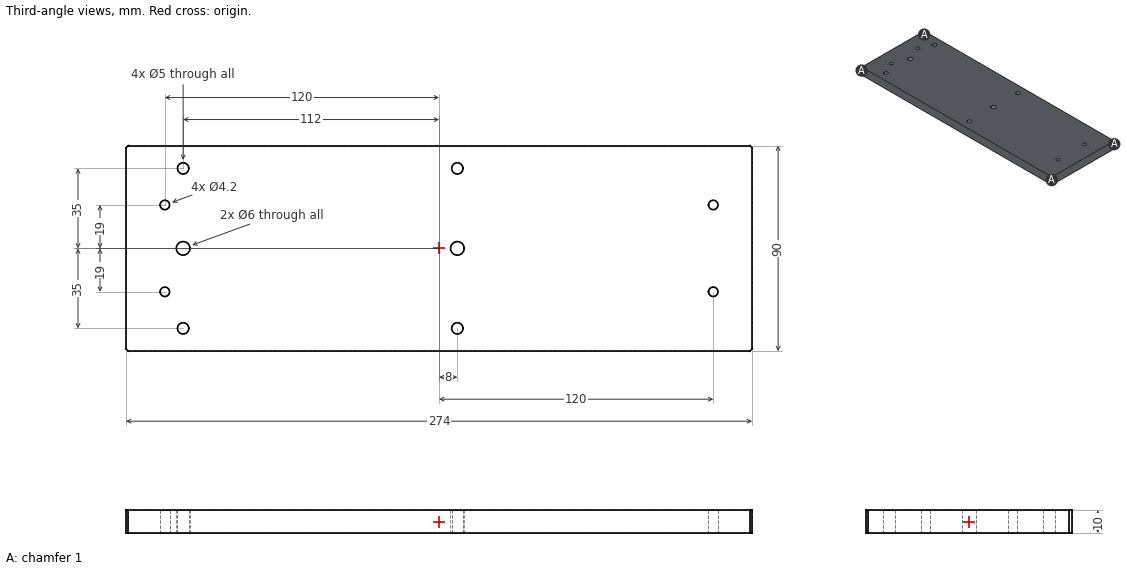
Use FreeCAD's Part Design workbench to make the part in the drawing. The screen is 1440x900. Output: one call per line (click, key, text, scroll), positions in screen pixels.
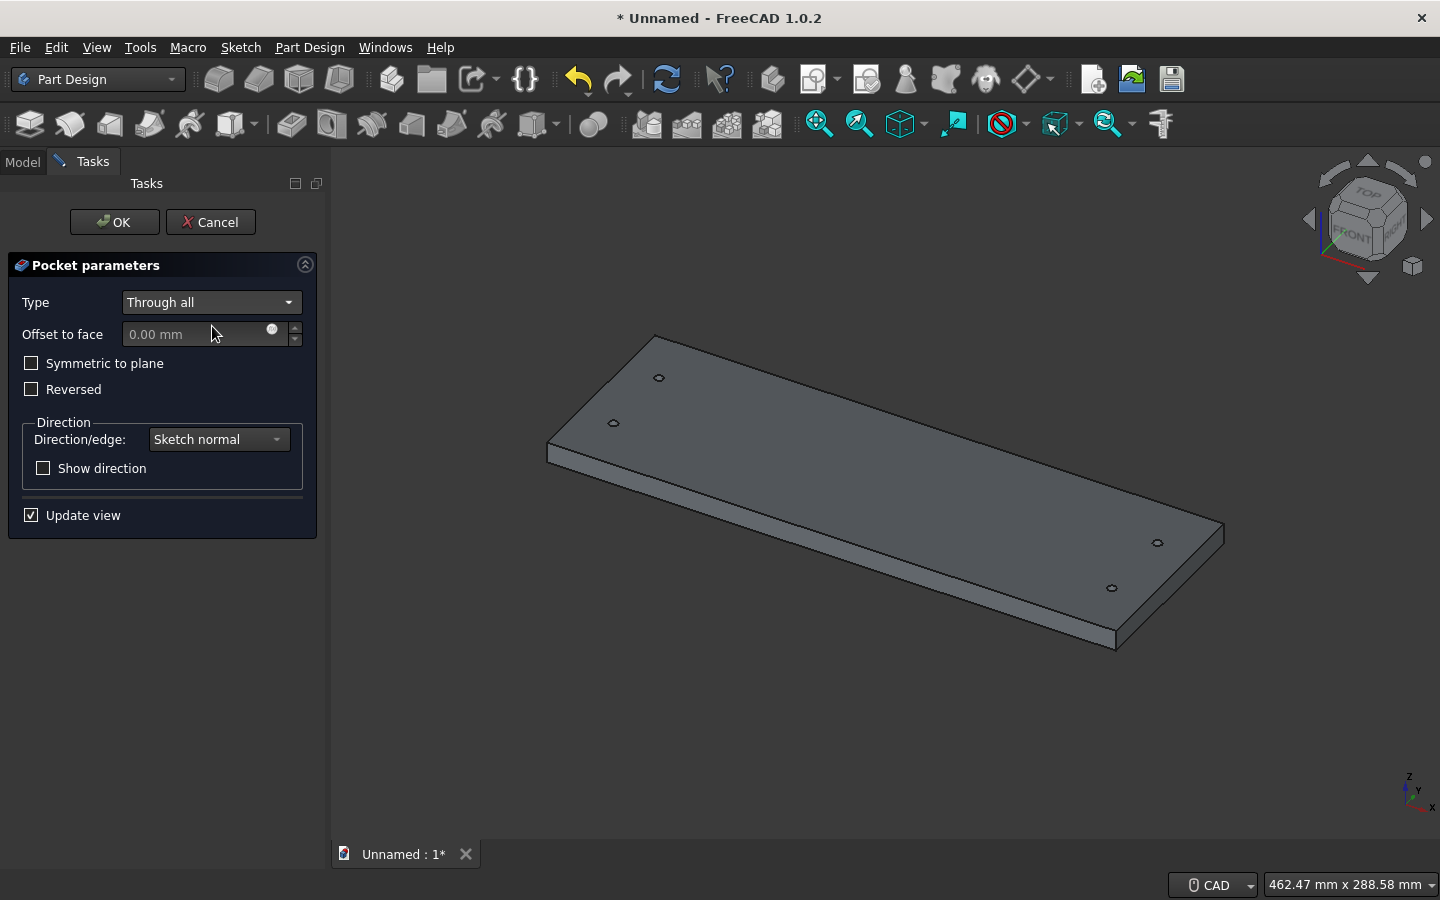
click(115, 222)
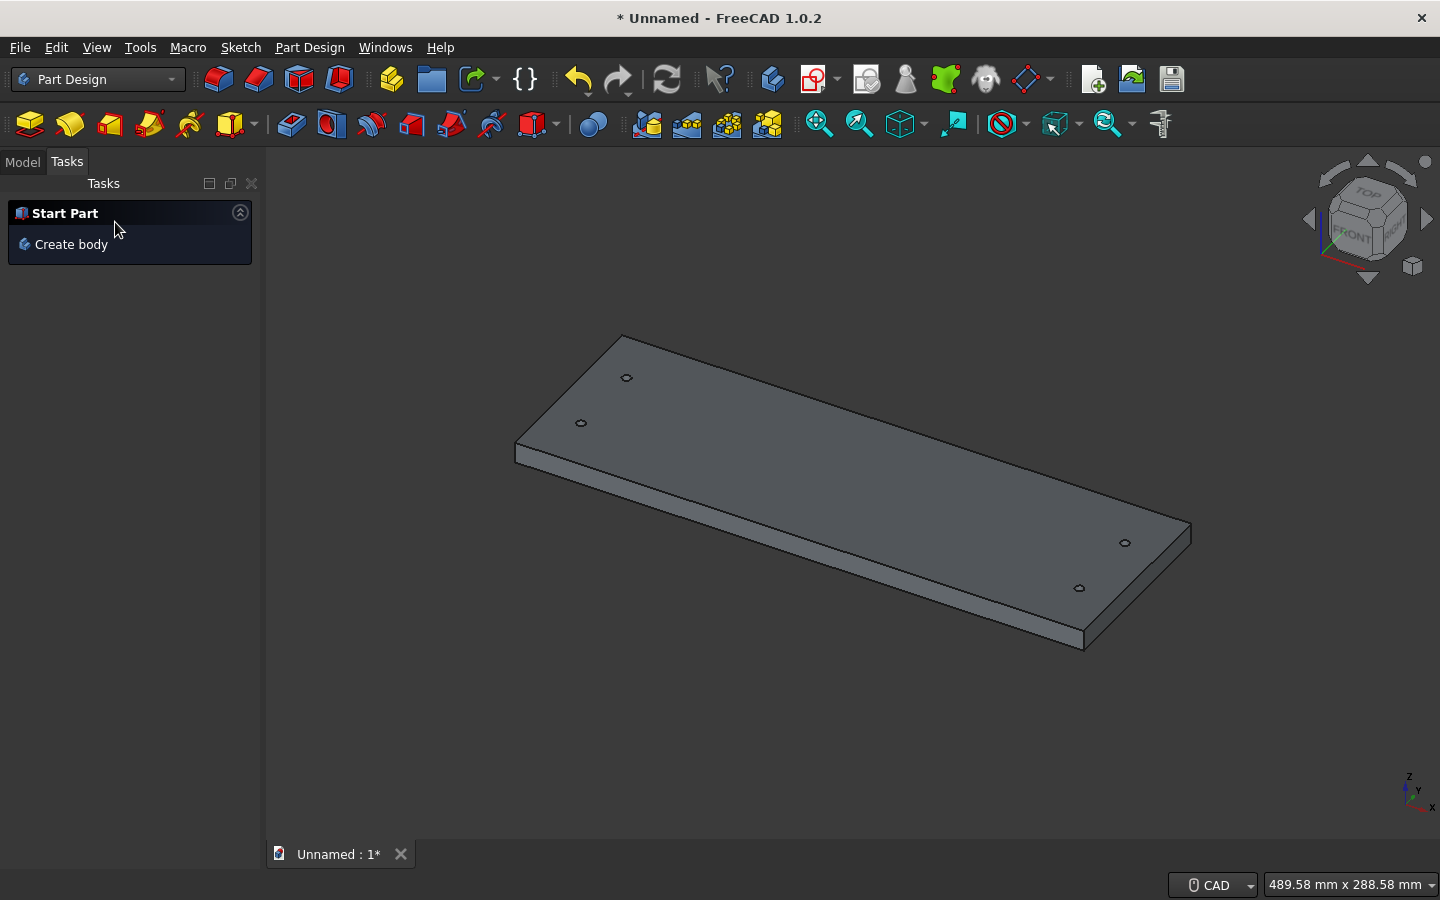
key(5)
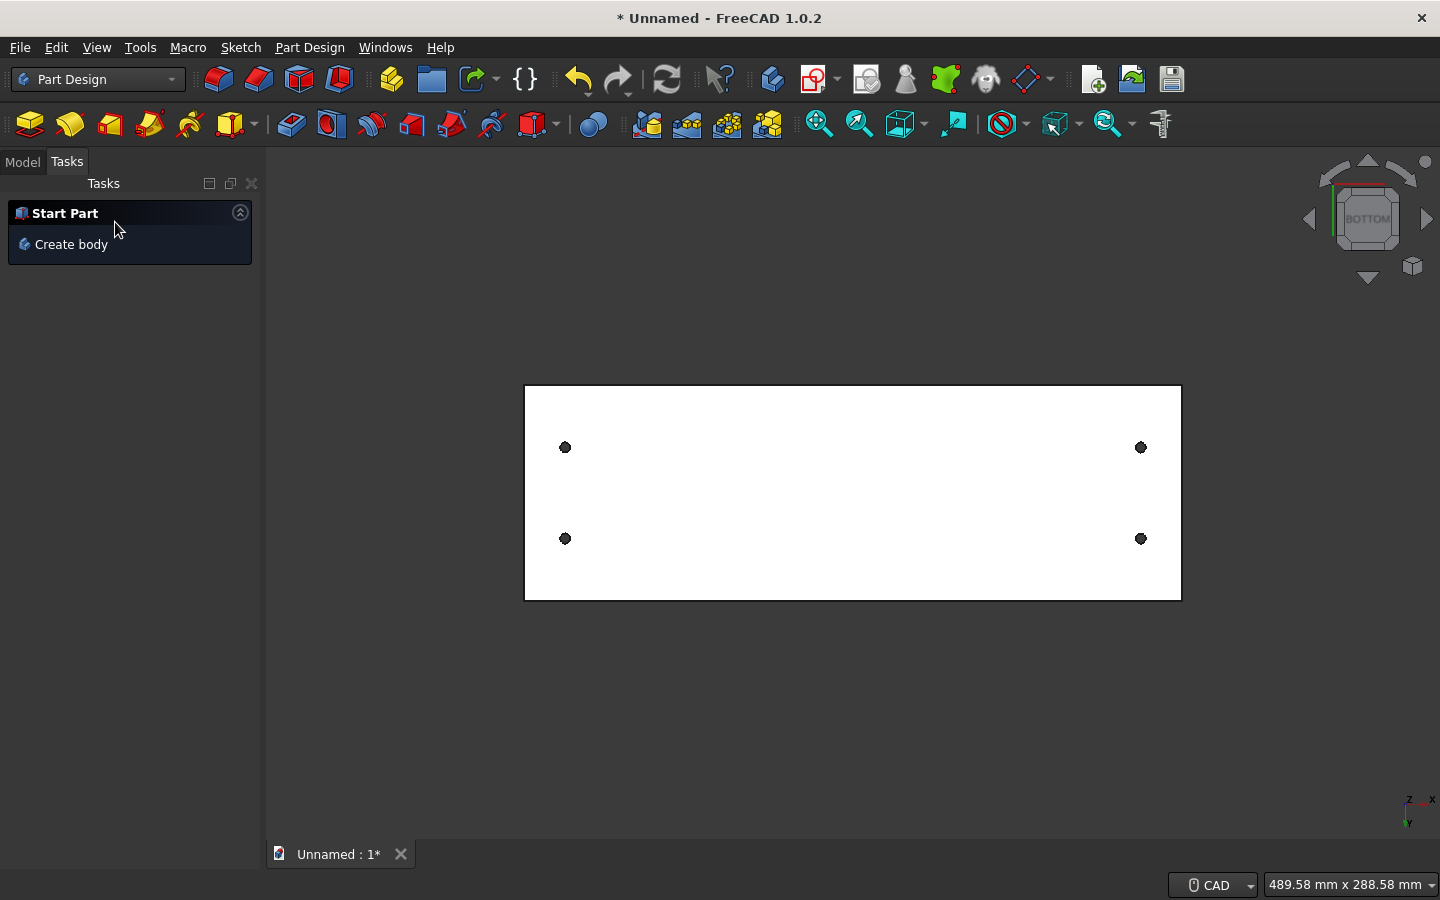
click(947, 492)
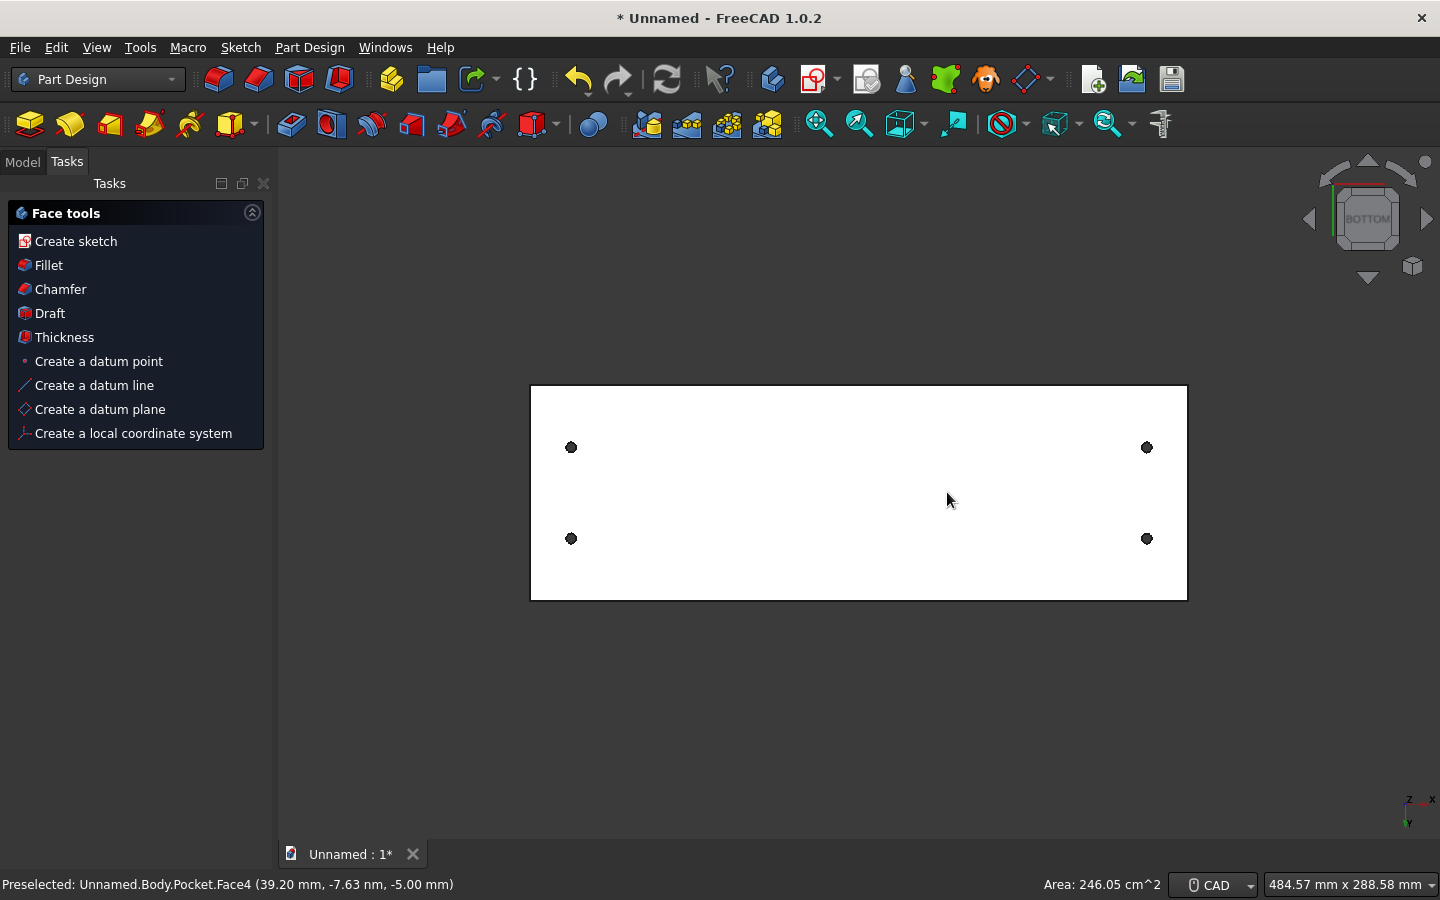
click(814, 80)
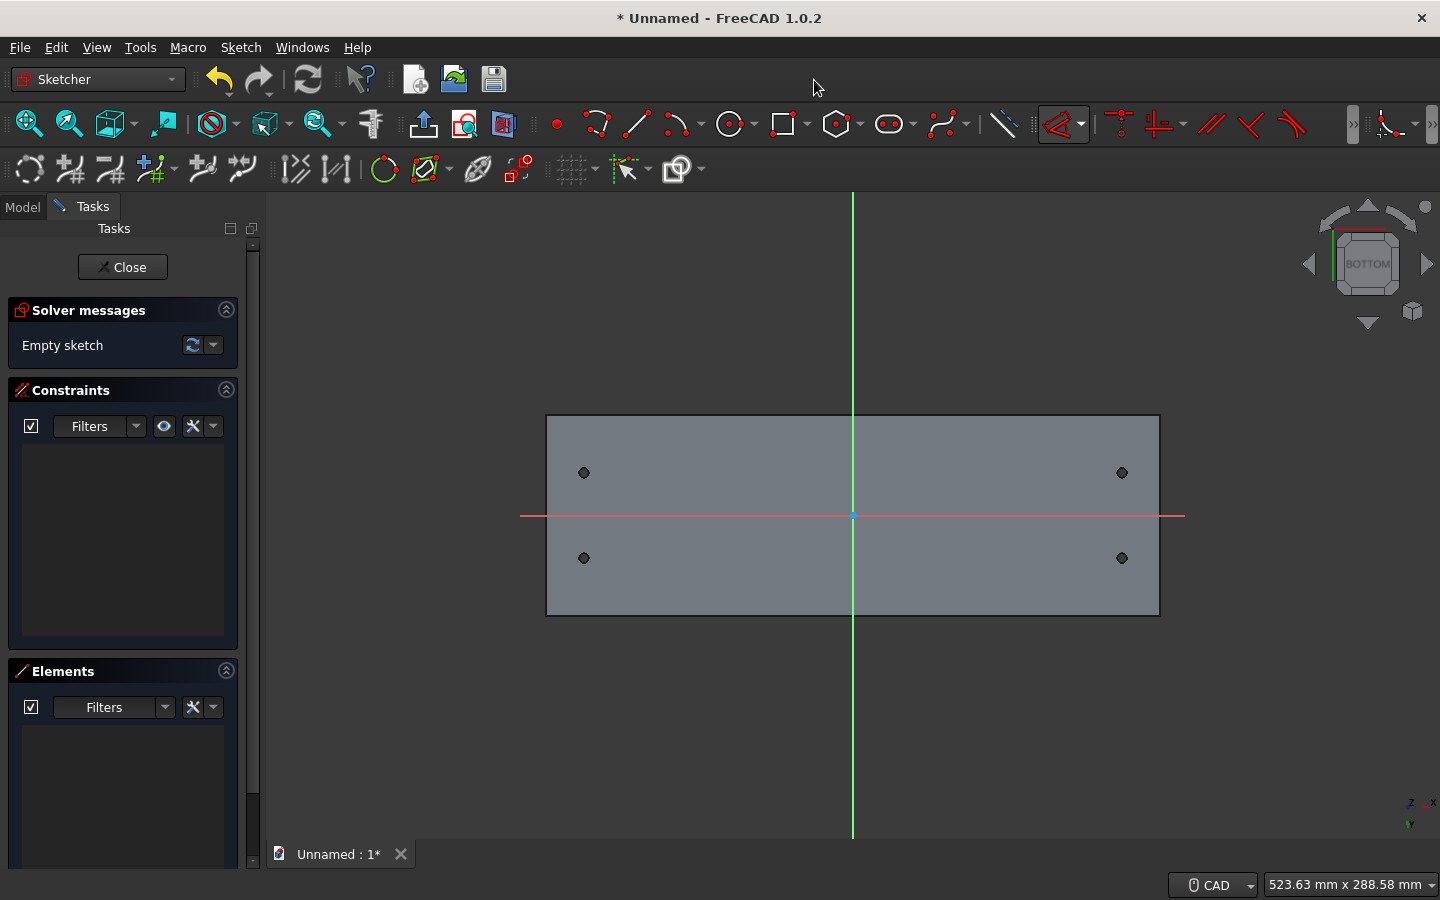
scroll(708, 516, up, 5)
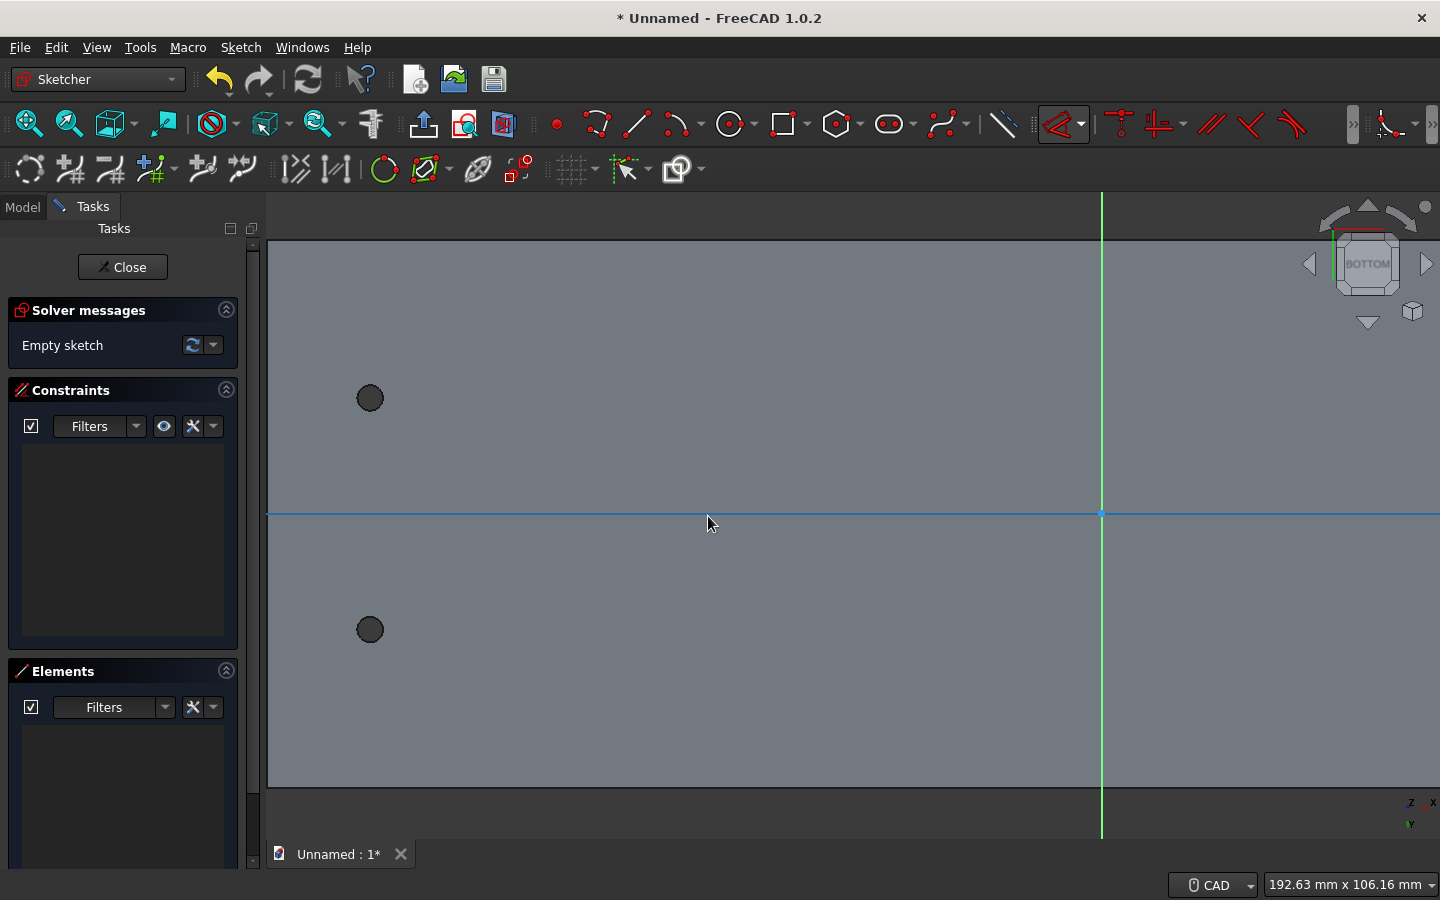
key(g)
key(c)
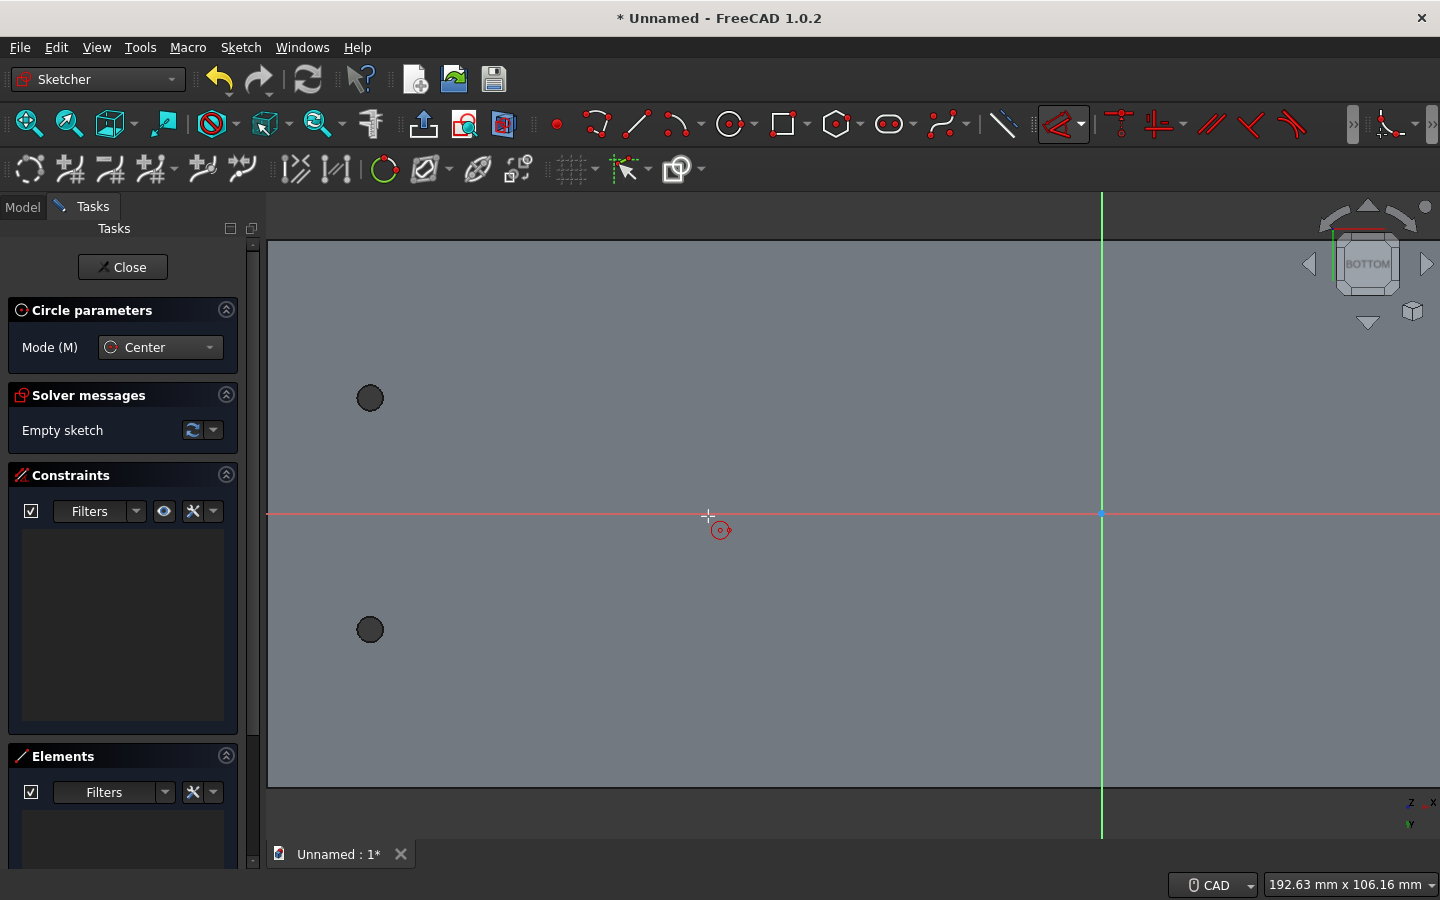
scroll(419, 727, up, 2)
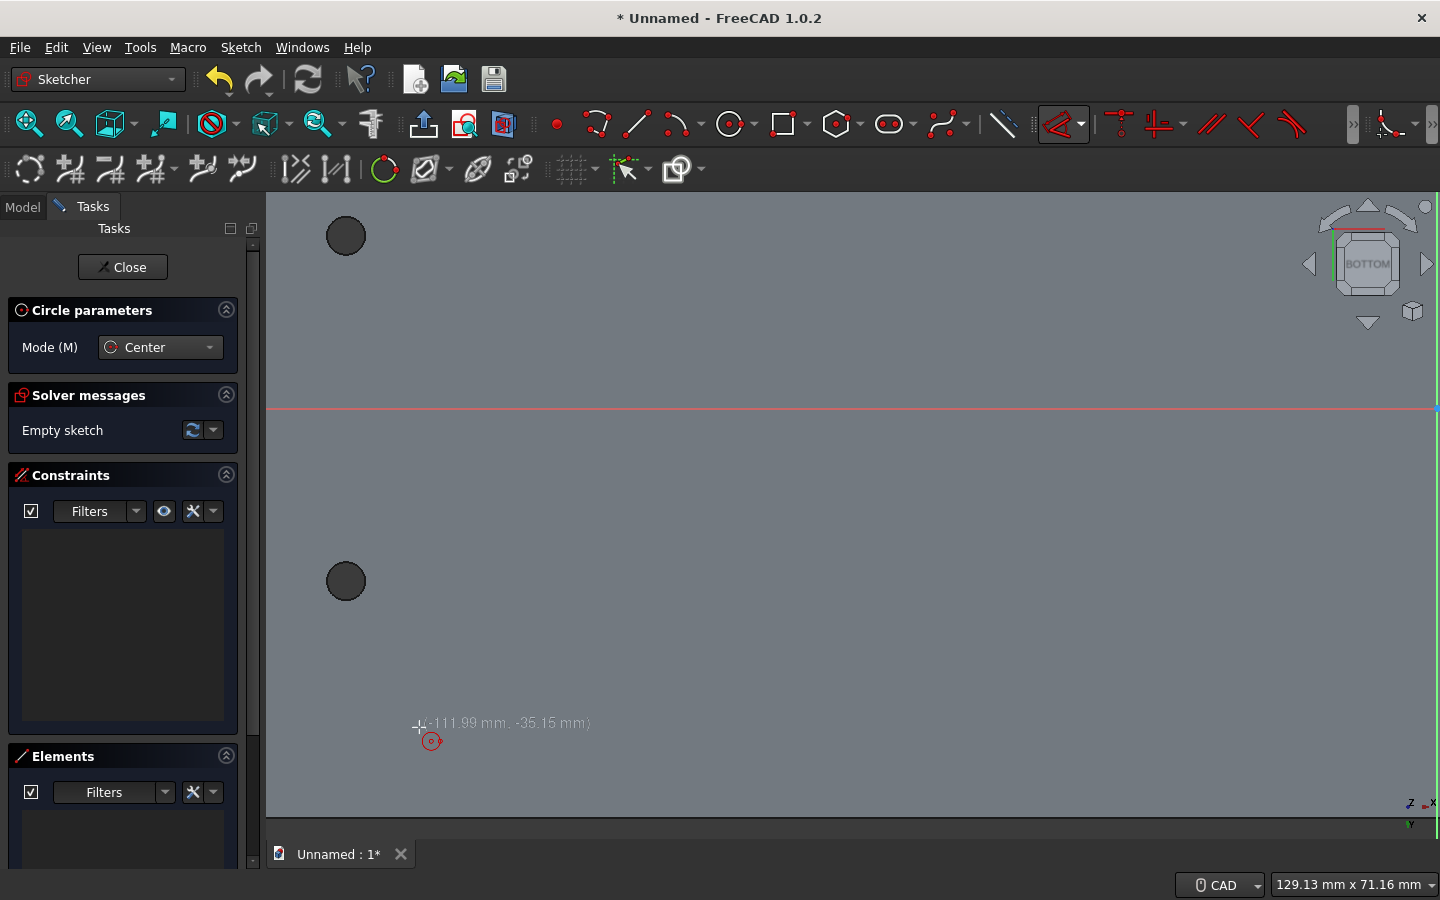
click(419, 727)
click(435, 711)